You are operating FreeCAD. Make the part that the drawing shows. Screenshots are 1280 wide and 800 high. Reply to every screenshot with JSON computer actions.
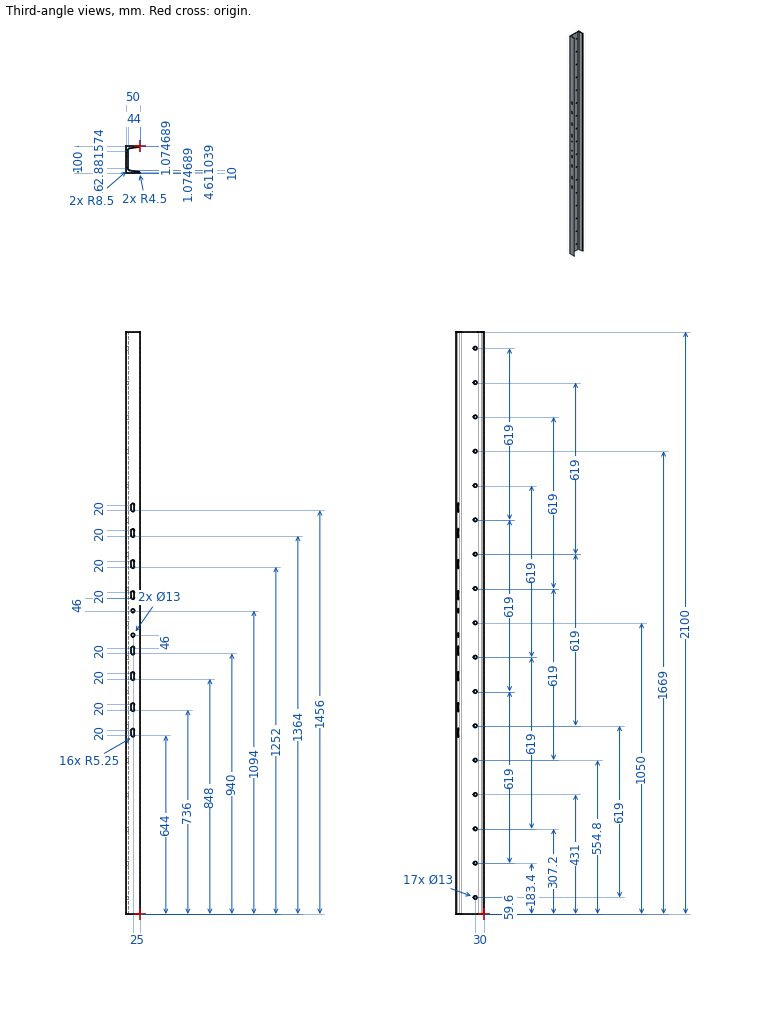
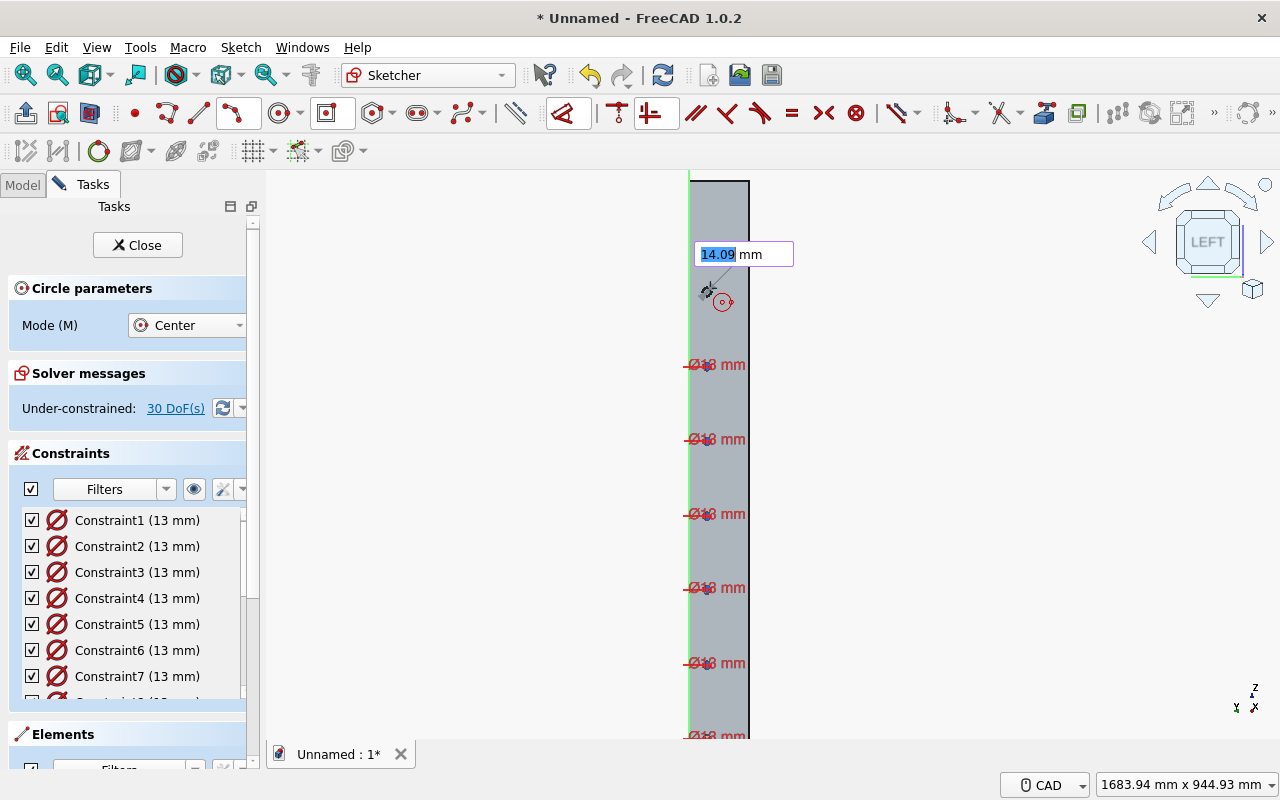
{"action": "type", "text": "13"}
{"action": "key", "text": "Return"}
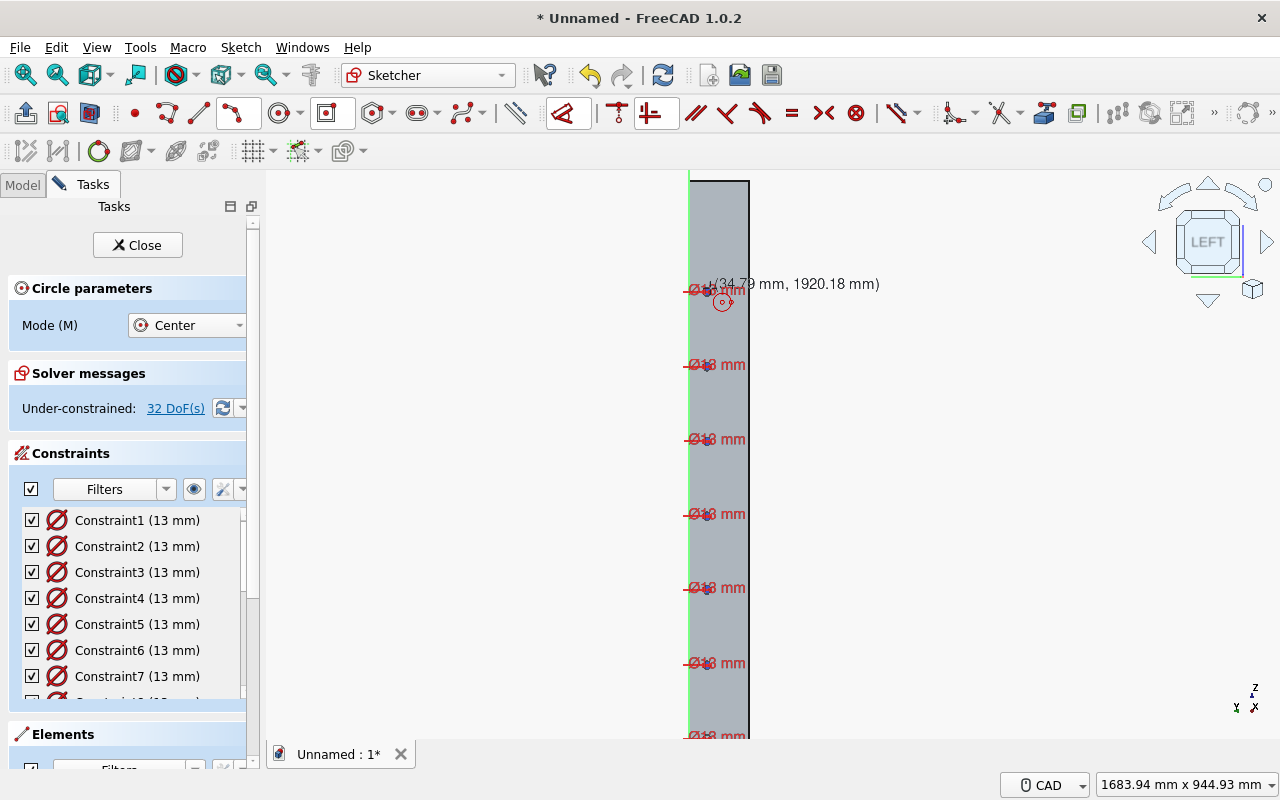
{"action": "scroll", "coordinate": [707, 217], "scroll_direction": "up", "scroll_amount": 9}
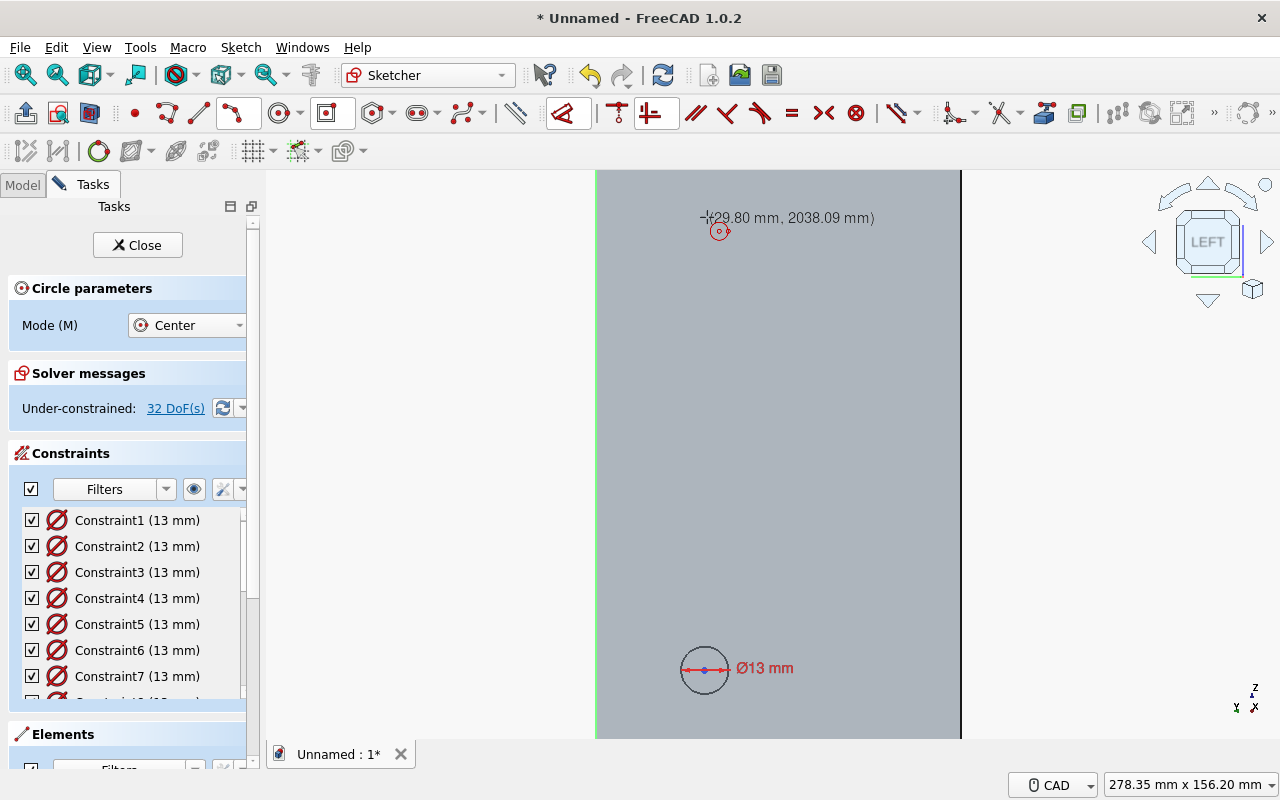
{"action": "scroll", "coordinate": [707, 273], "scroll_direction": "down", "scroll_amount": 15}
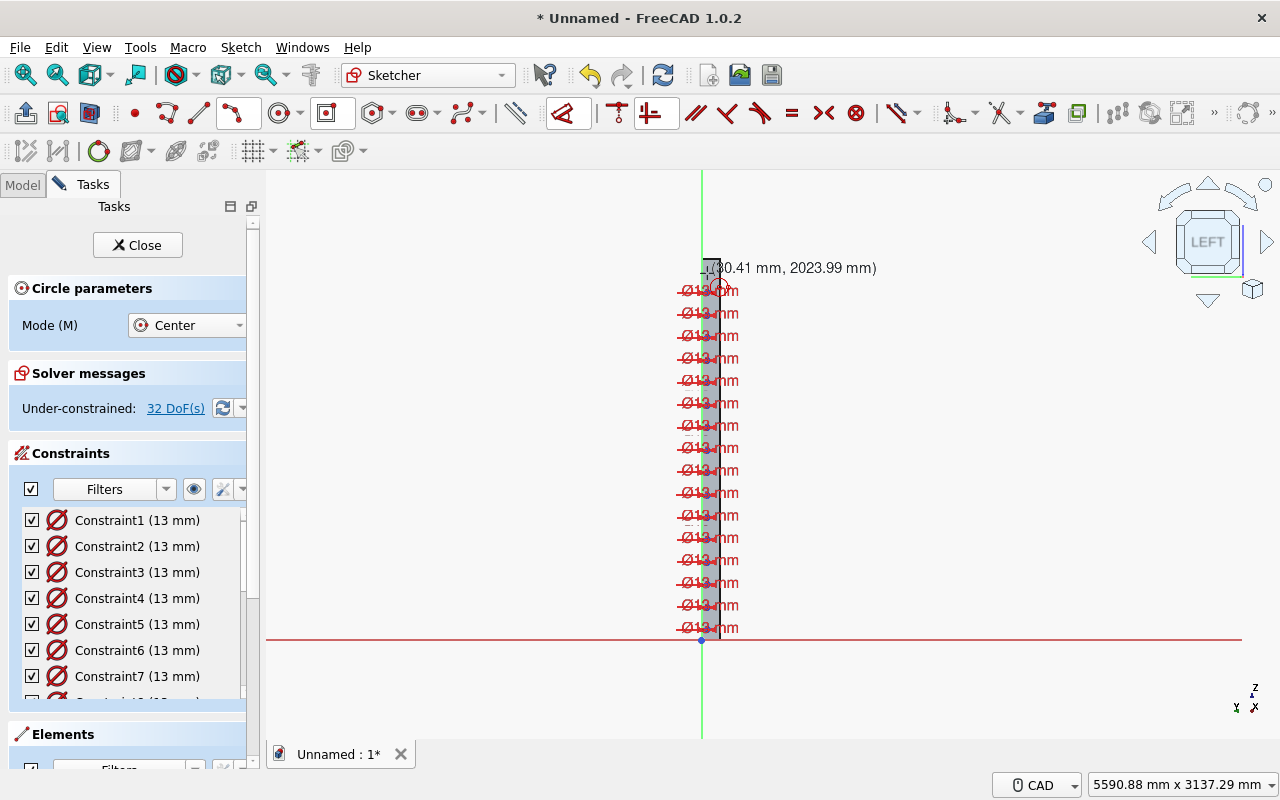
{"action": "scroll", "coordinate": [707, 270], "scroll_direction": "up", "scroll_amount": 6}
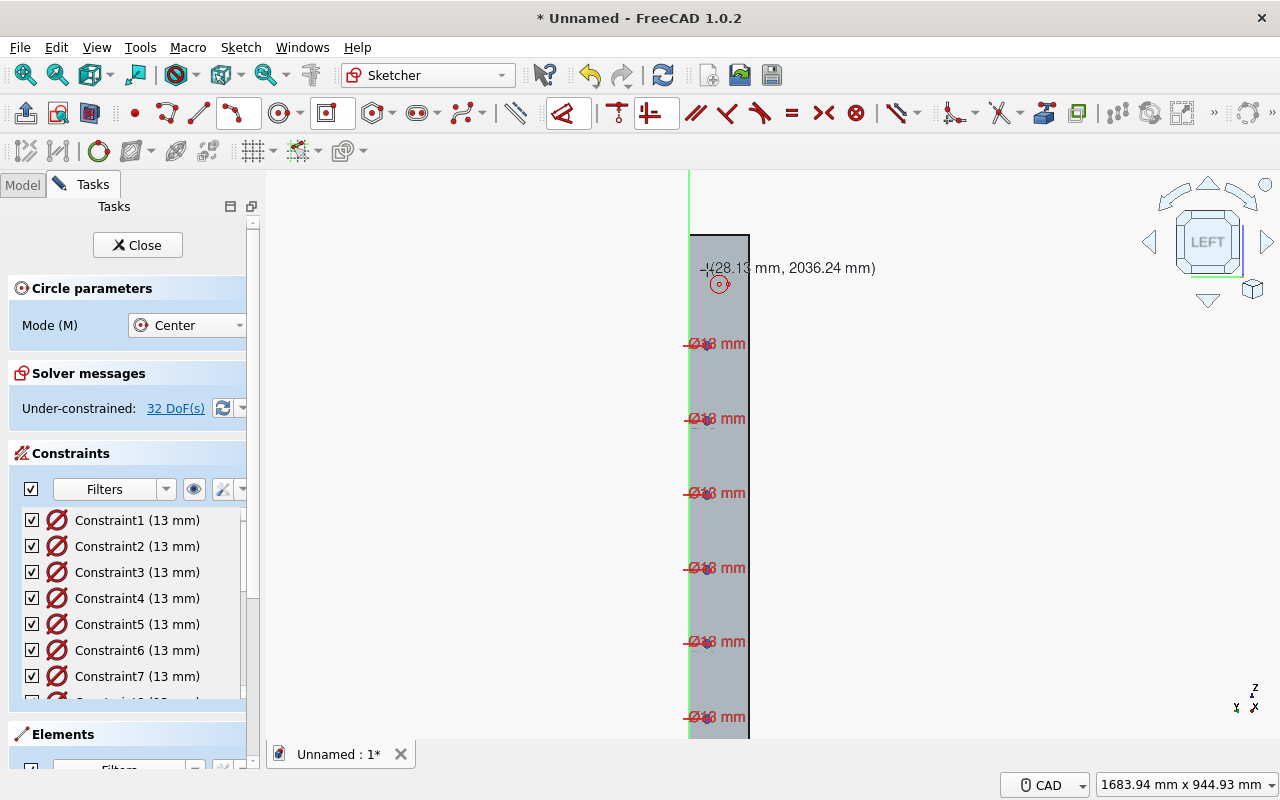
{"action": "left_click", "coordinate": [707, 270]}
{"action": "mouse_move", "coordinate": [710, 268]}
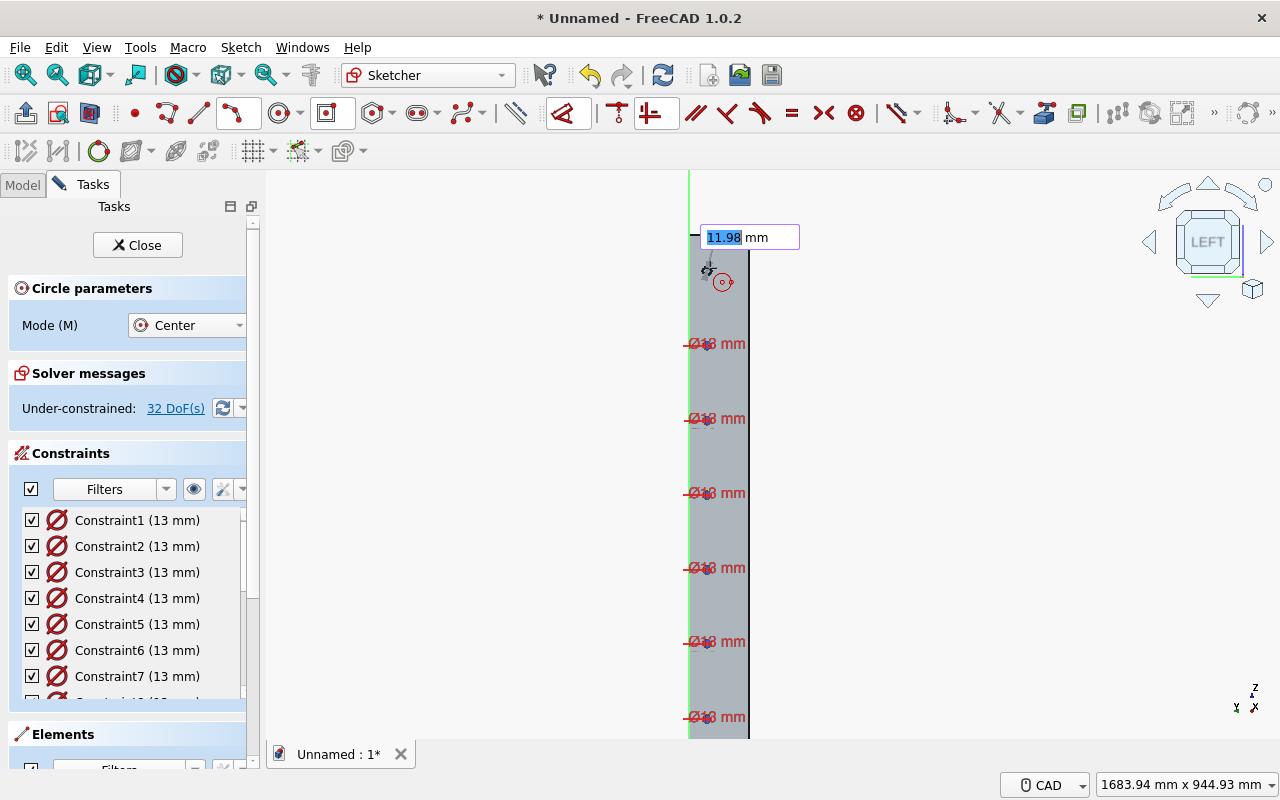
{"action": "type", "text": "13"}
{"action": "key", "text": "Return"}
{"action": "key", "text": "Escape"}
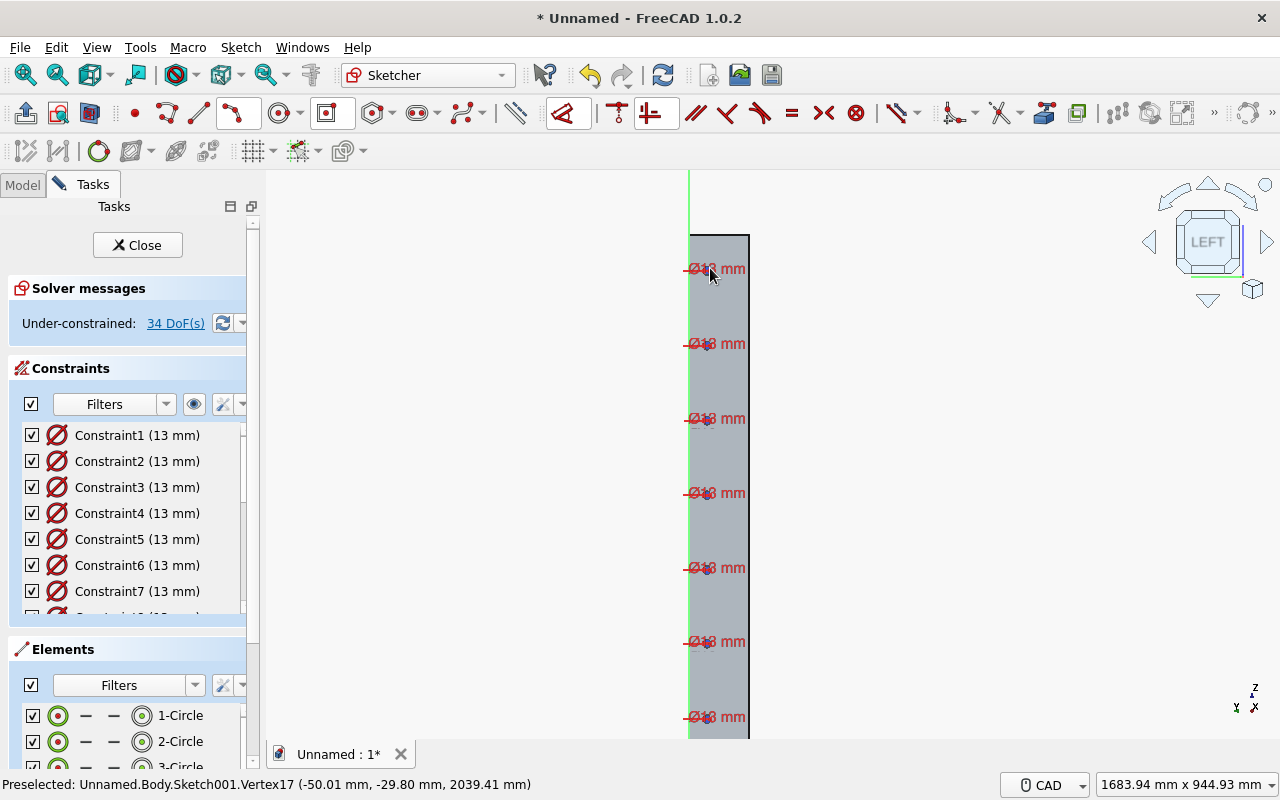
{"action": "scroll", "coordinate": [706, 270], "scroll_direction": "down", "scroll_amount": 6}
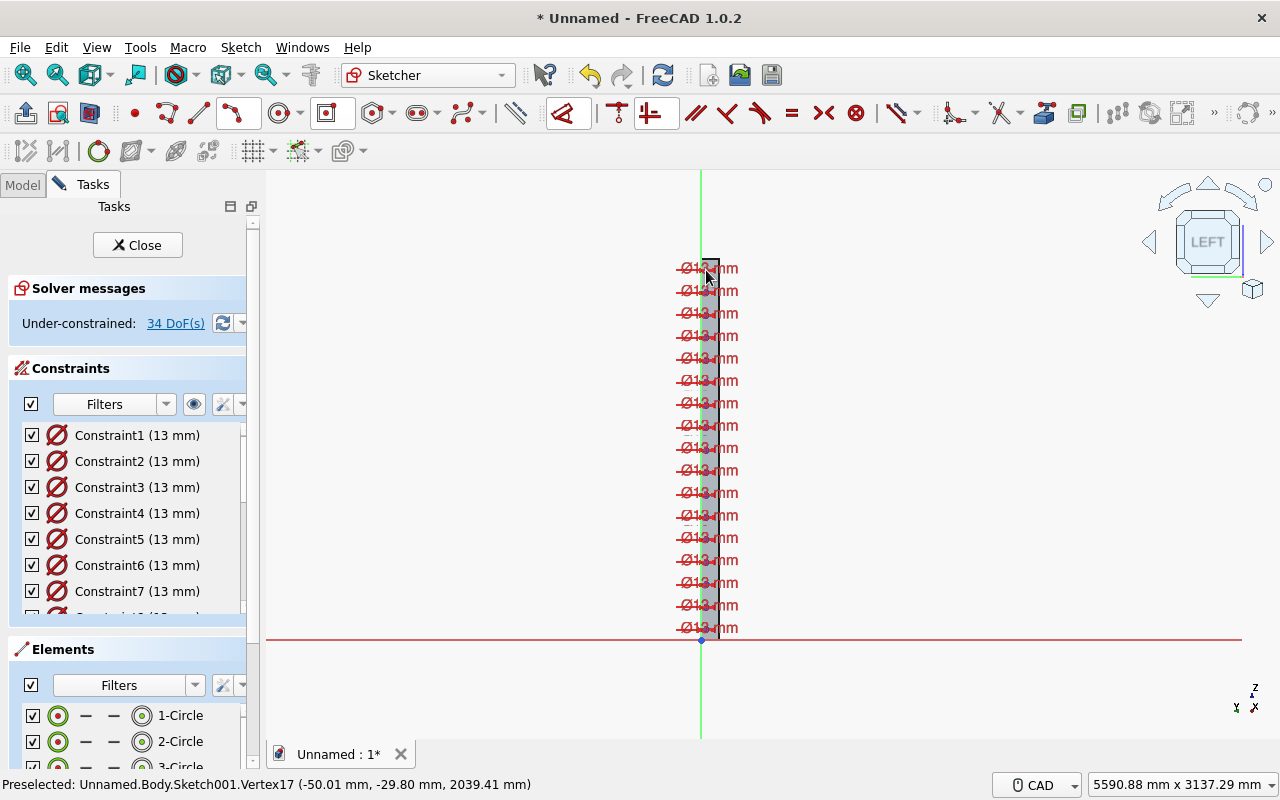
{"action": "left_click", "coordinate": [707, 630]}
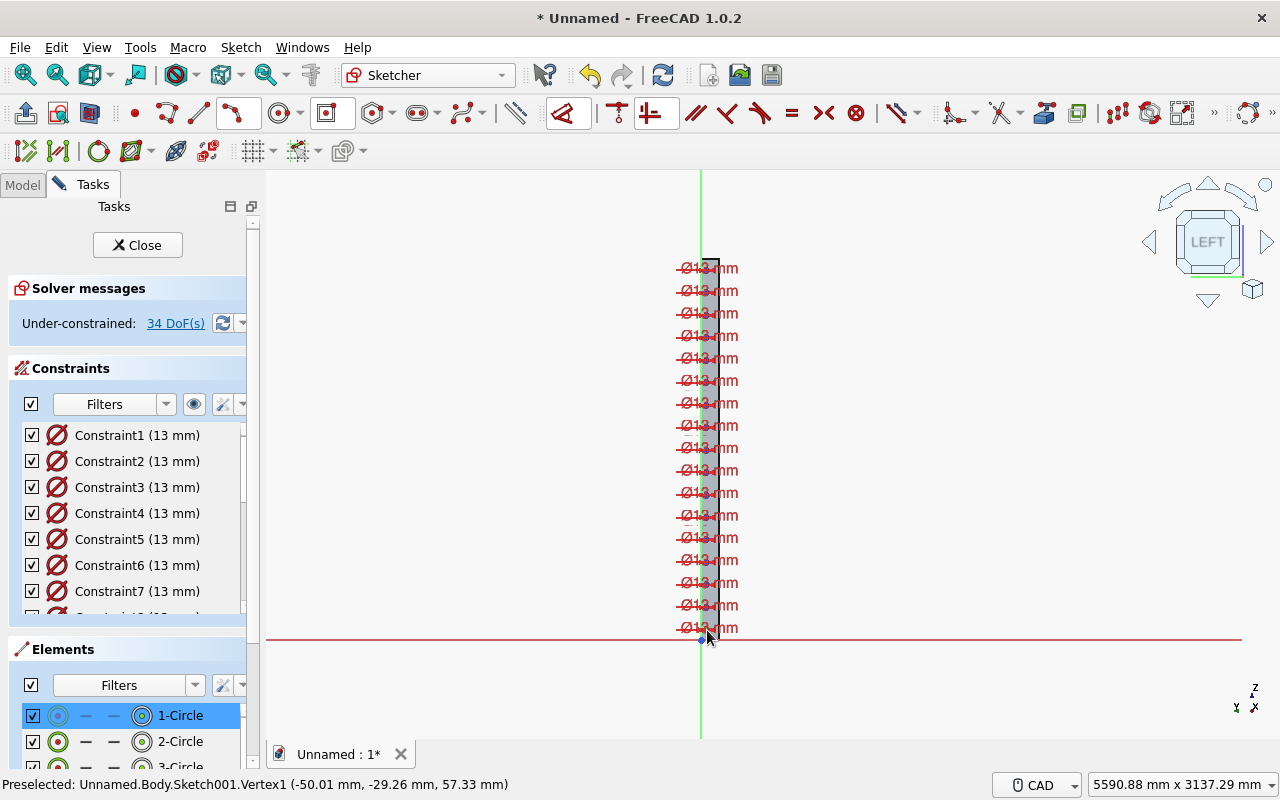
{"action": "left_click", "coordinate": [707, 607]}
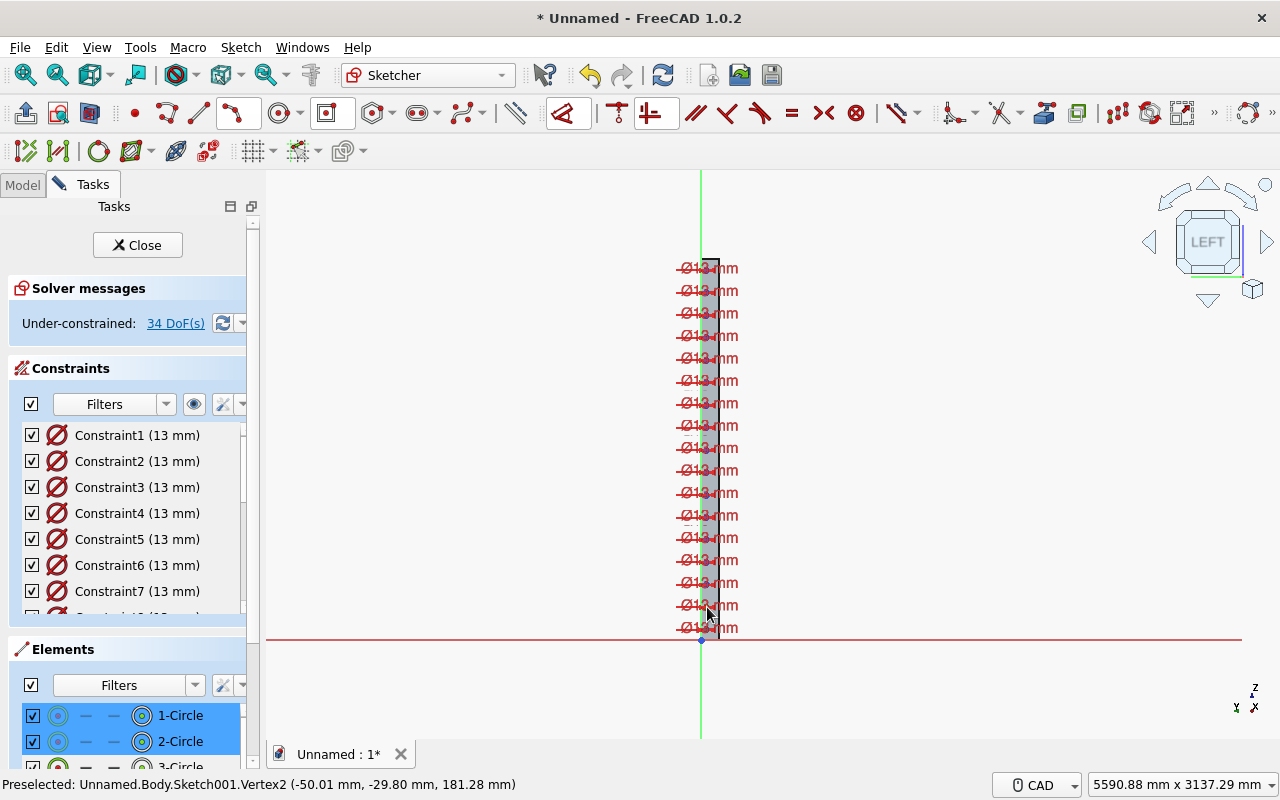
{"action": "key", "text": "v"}